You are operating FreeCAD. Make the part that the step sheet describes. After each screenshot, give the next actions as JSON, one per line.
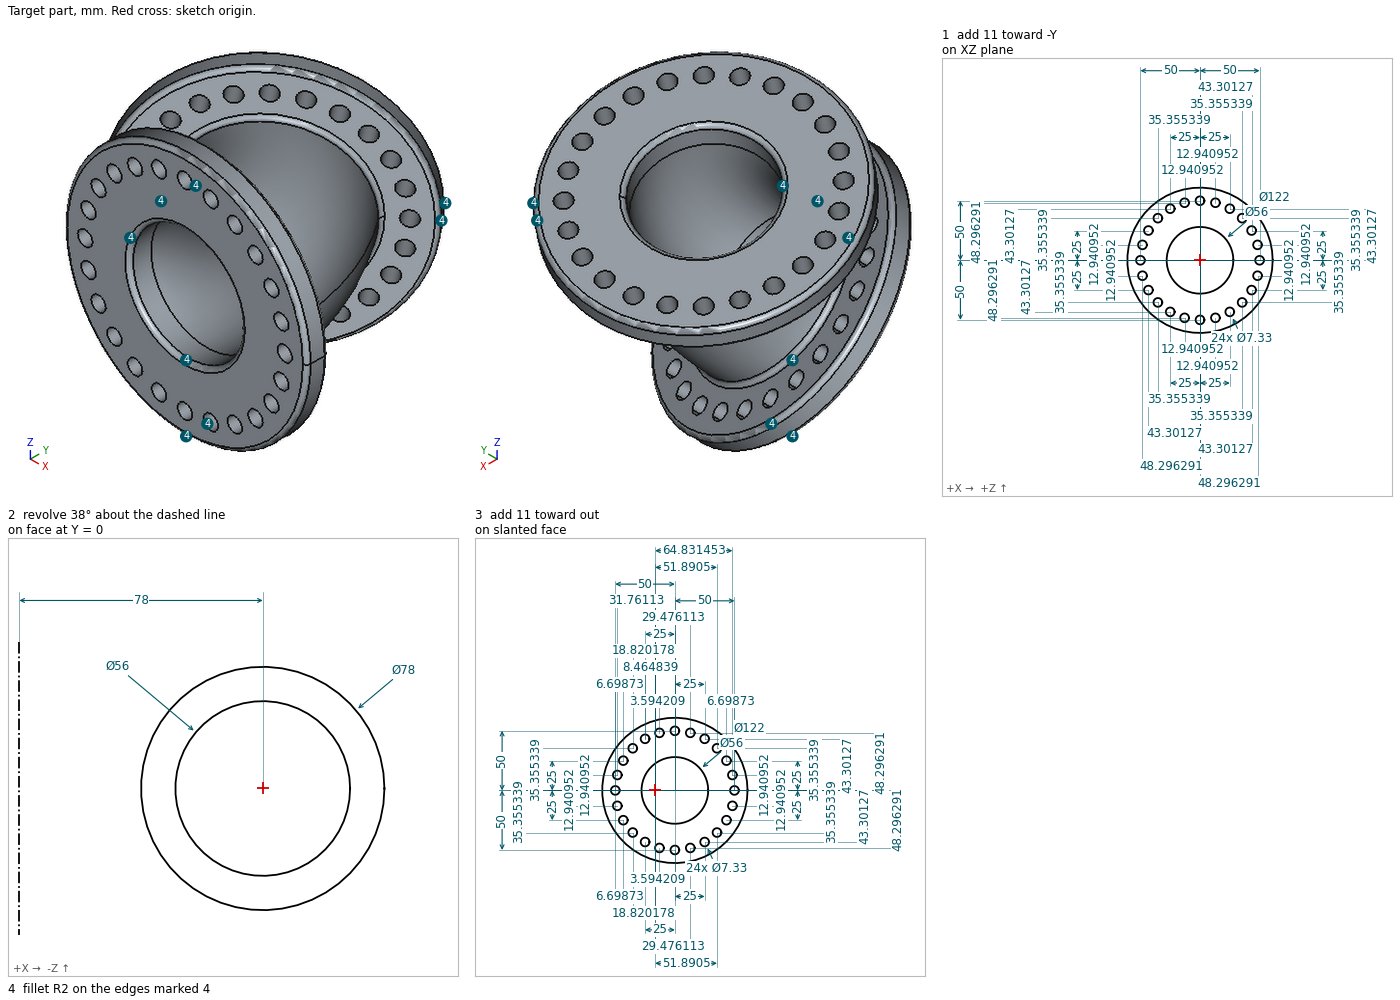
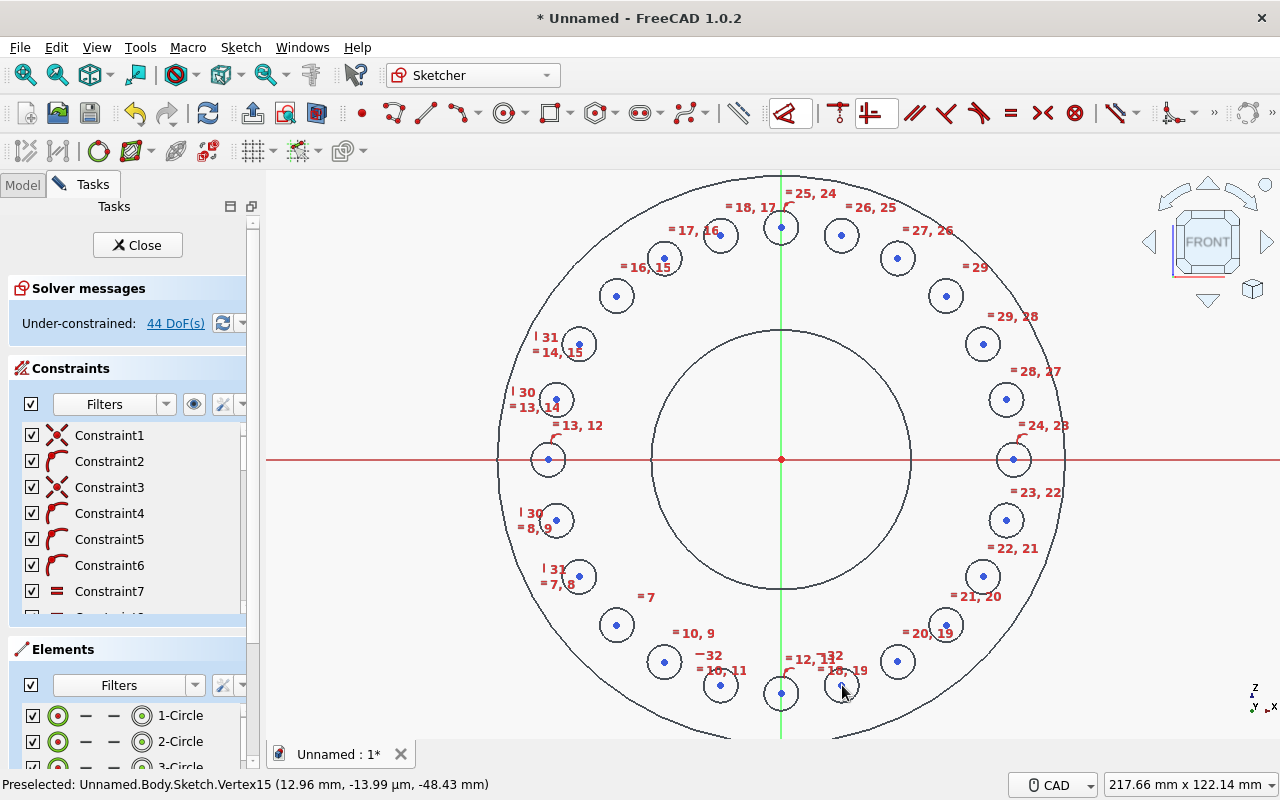
{"action": "left_click", "coordinate": [664, 662]}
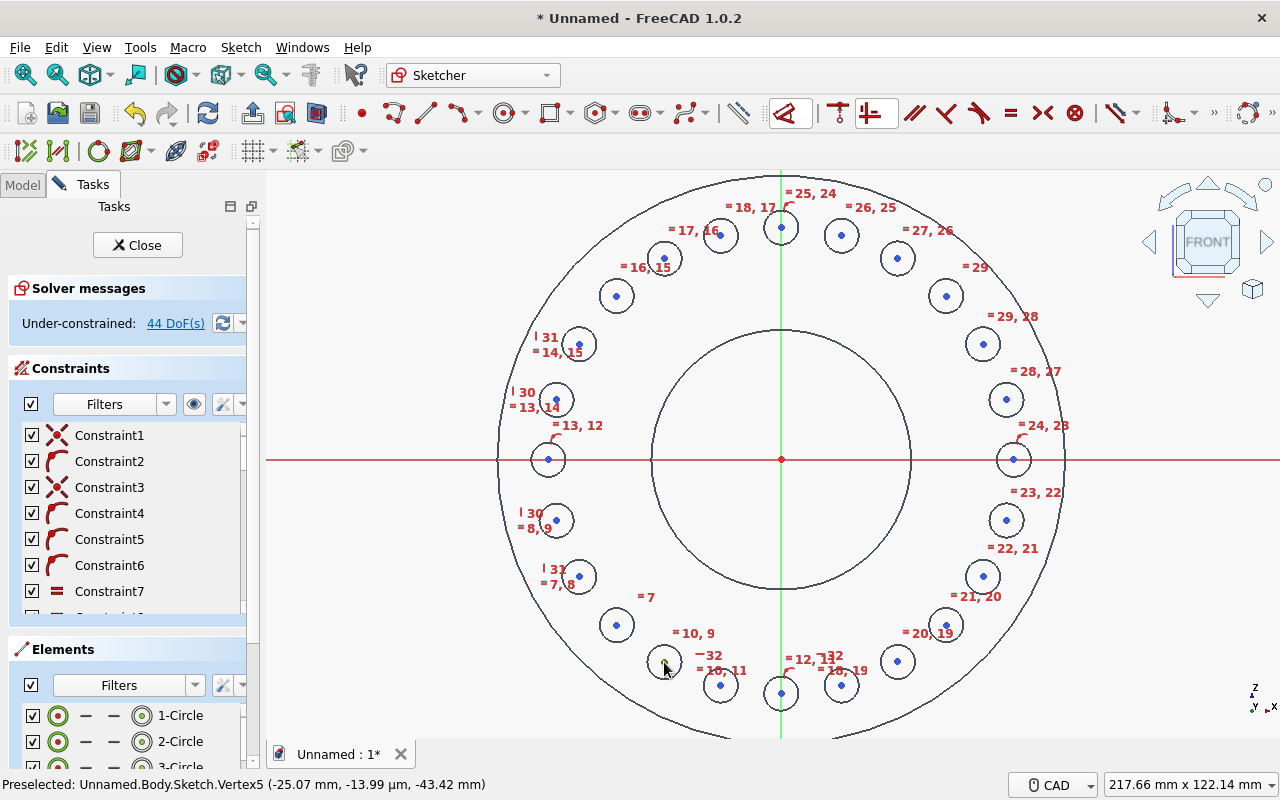
{"action": "left_click", "coordinate": [898, 662]}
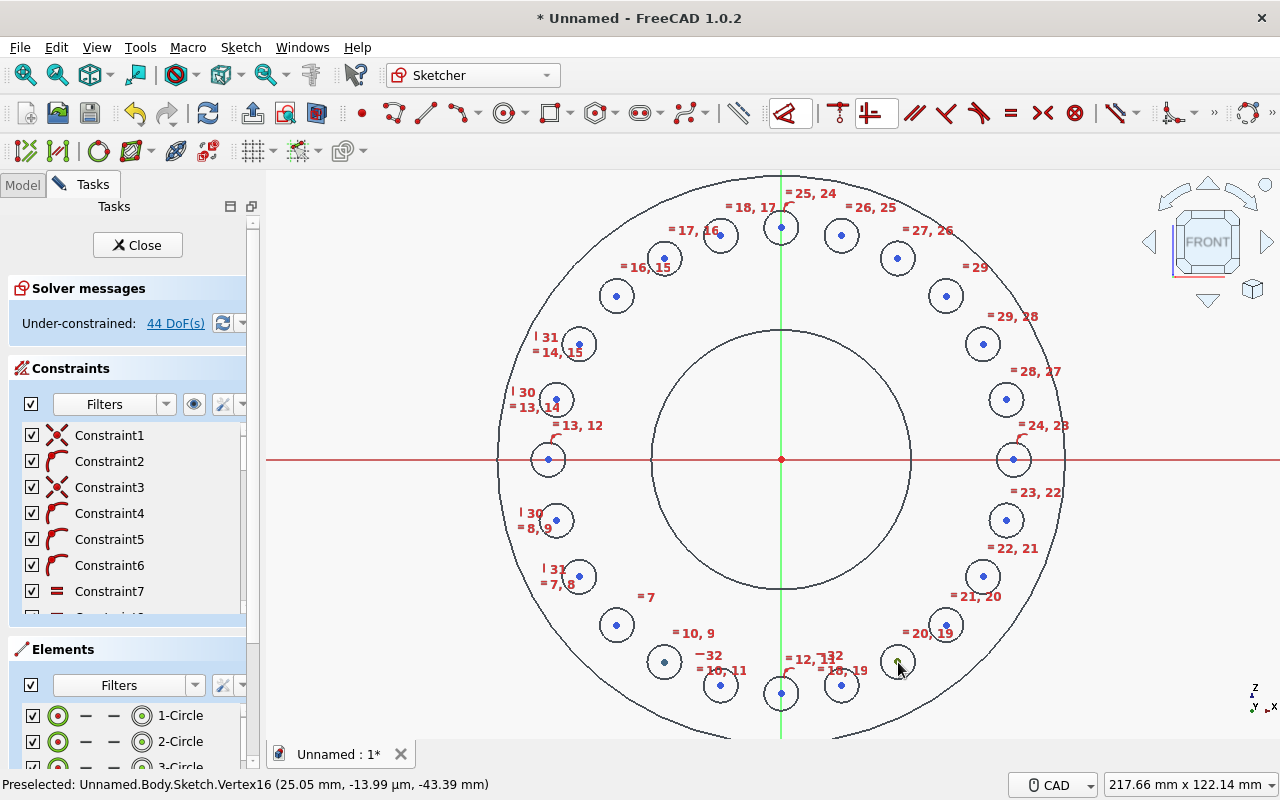
{"action": "key", "text": "h"}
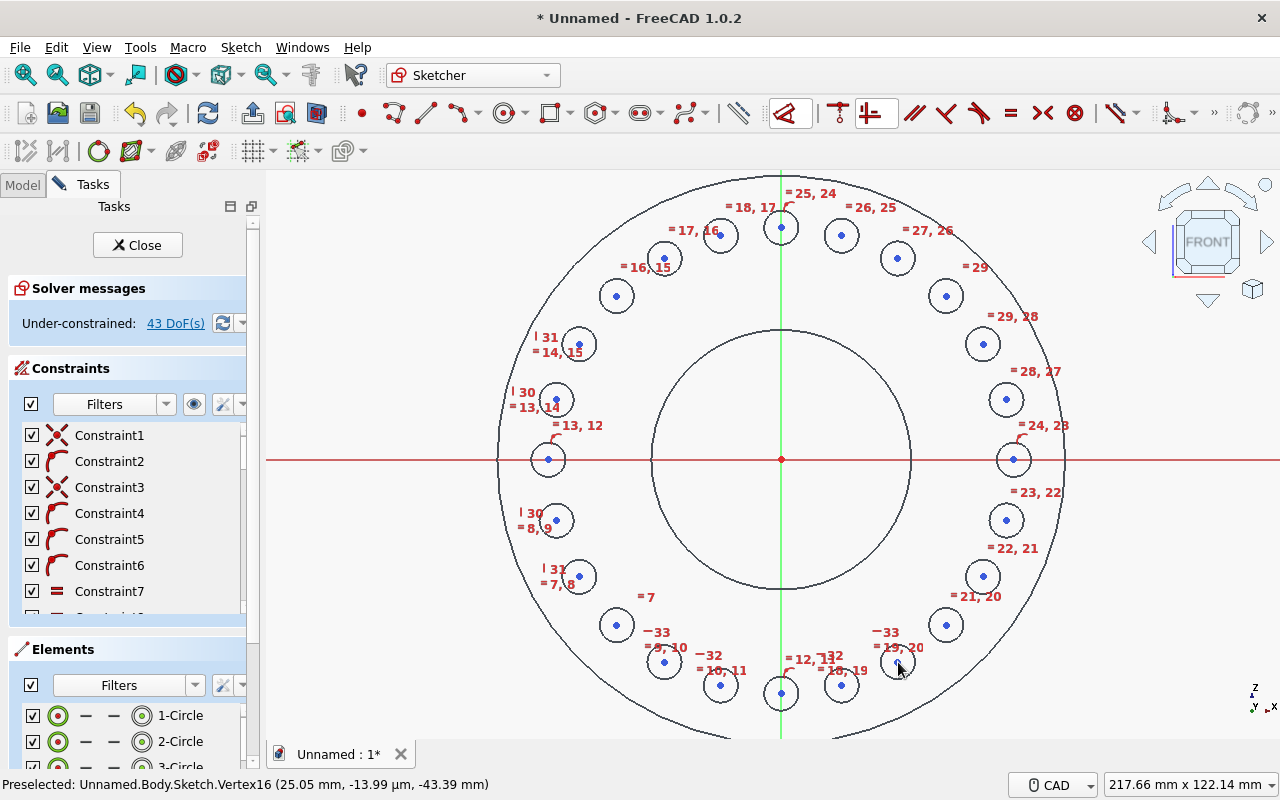
{"action": "left_click", "coordinate": [721, 236]}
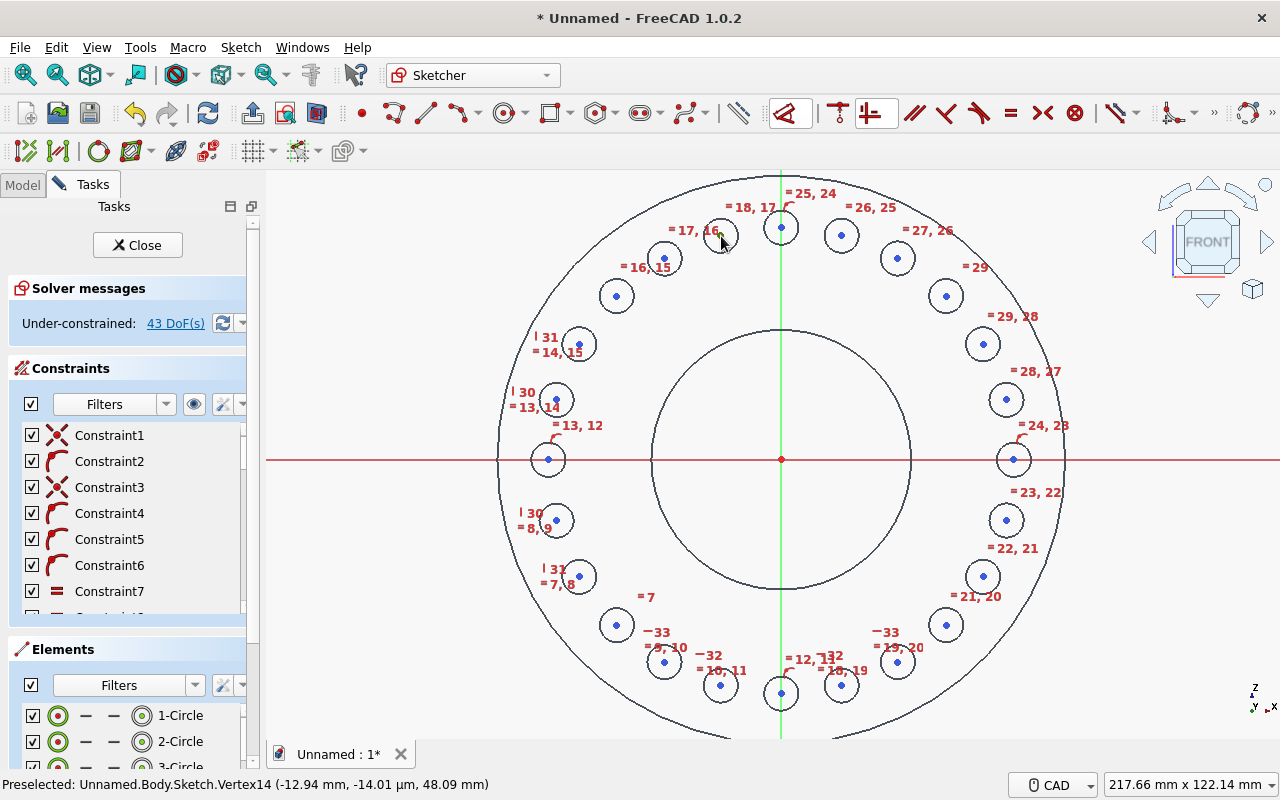
{"action": "left_click", "coordinate": [842, 236]}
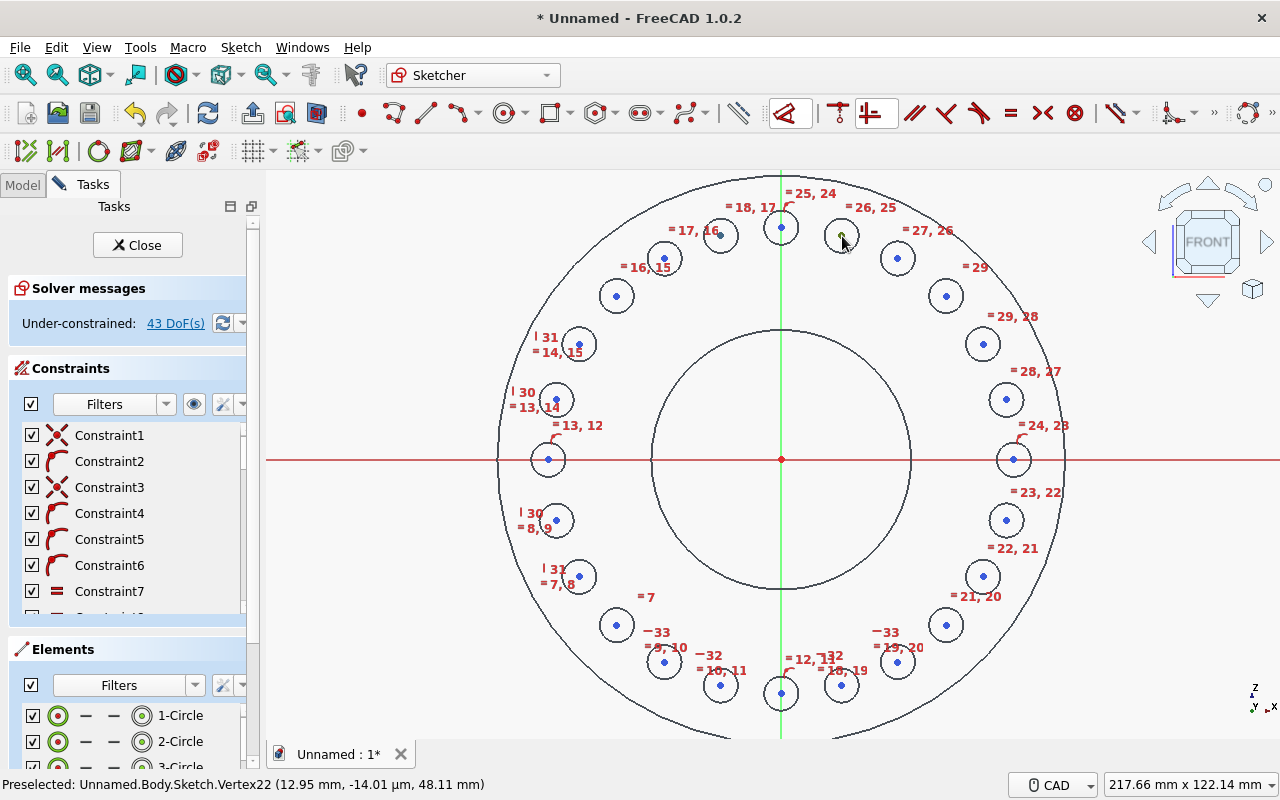
{"action": "left_click", "coordinate": [892, 114]}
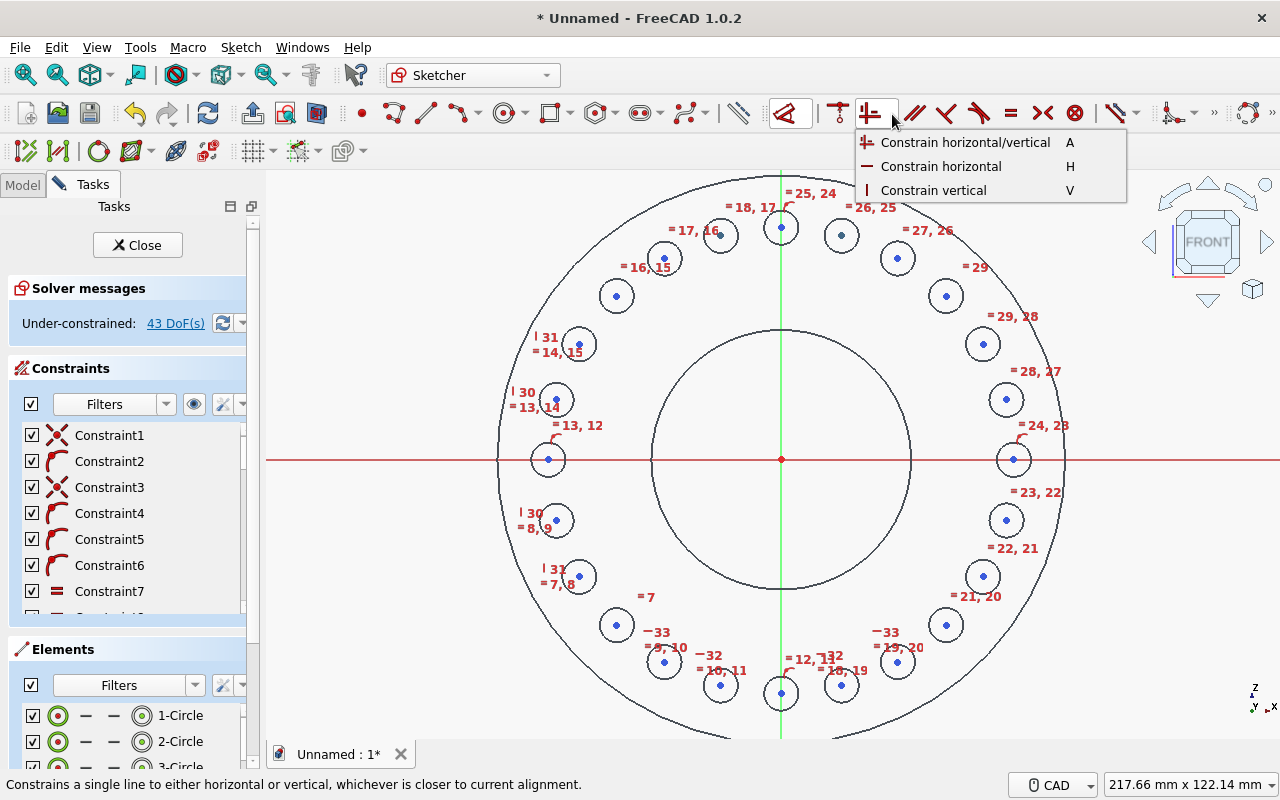
{"action": "left_click", "coordinate": [991, 166]}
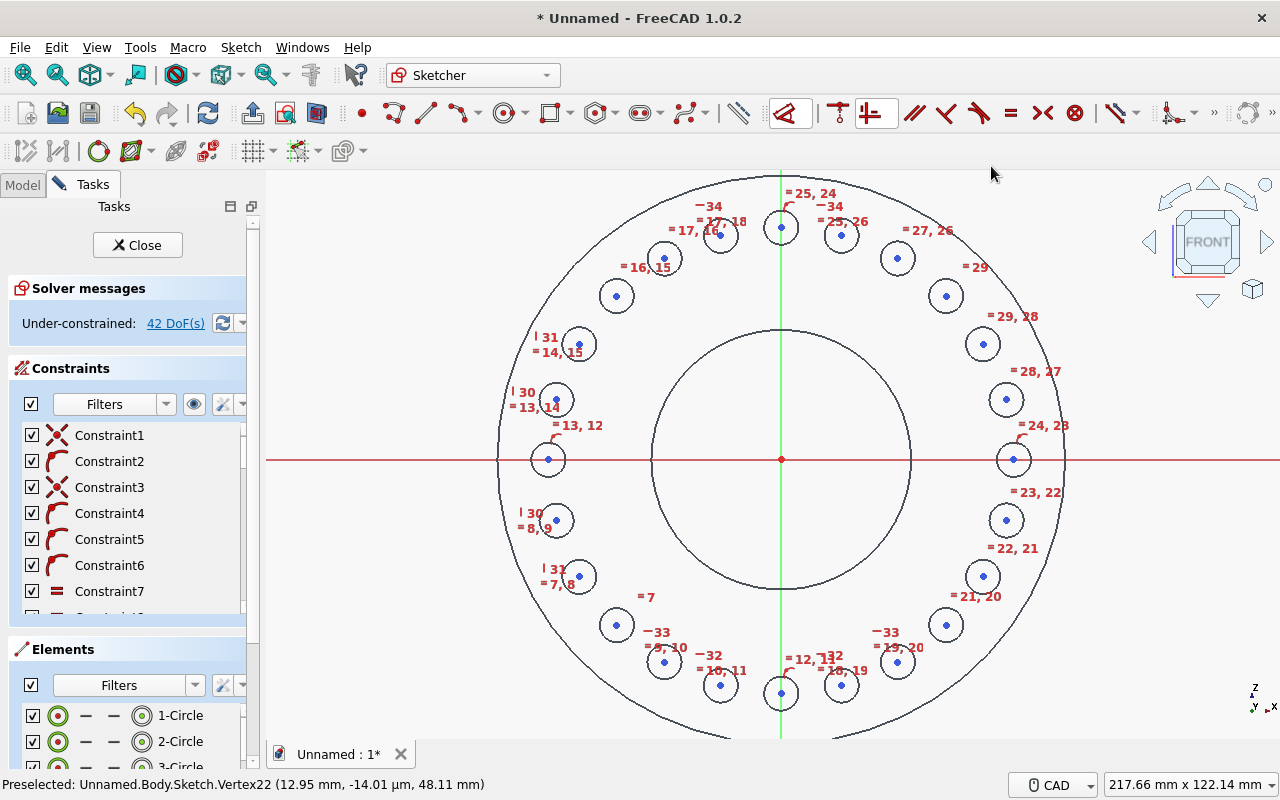
{"action": "left_click", "coordinate": [1007, 520]}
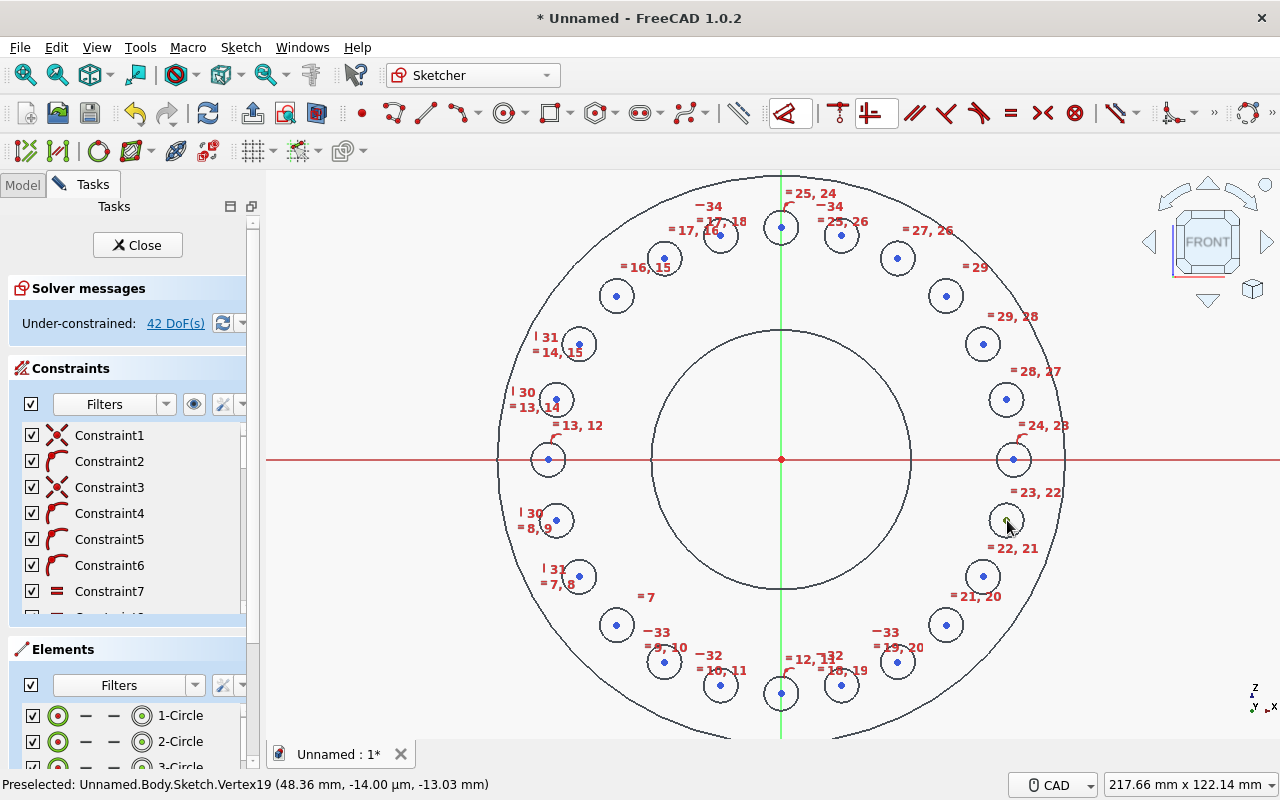
{"action": "left_click", "coordinate": [1007, 400]}